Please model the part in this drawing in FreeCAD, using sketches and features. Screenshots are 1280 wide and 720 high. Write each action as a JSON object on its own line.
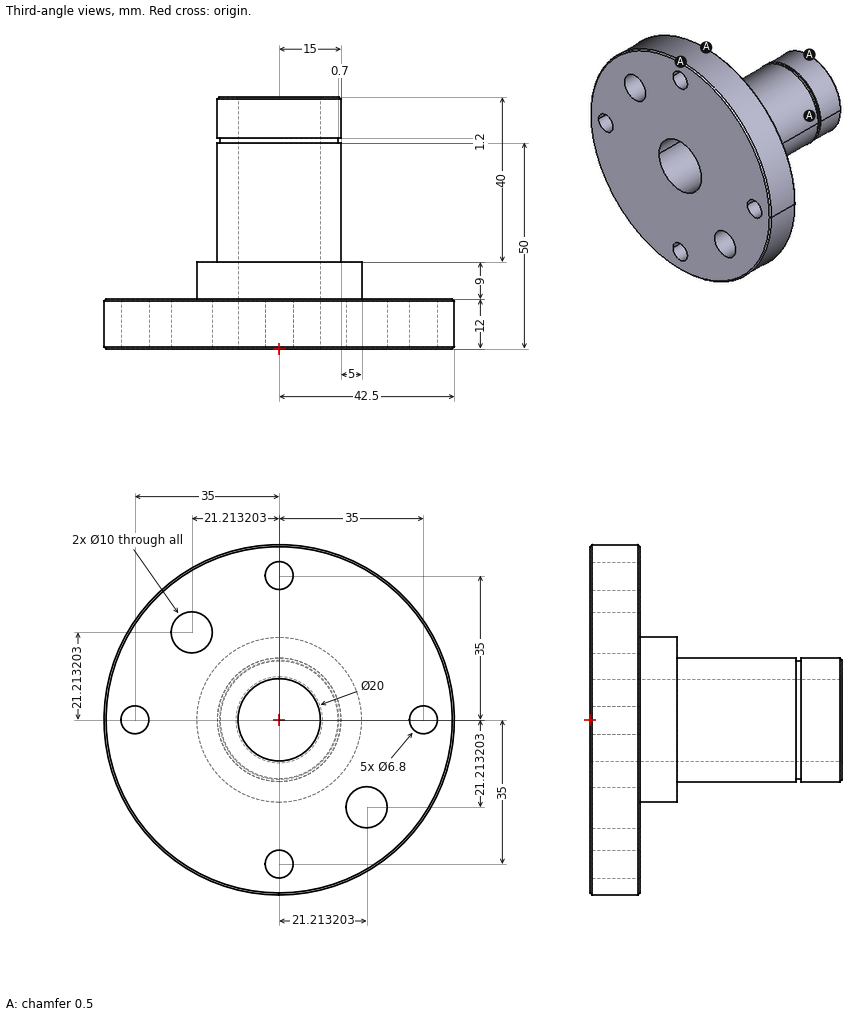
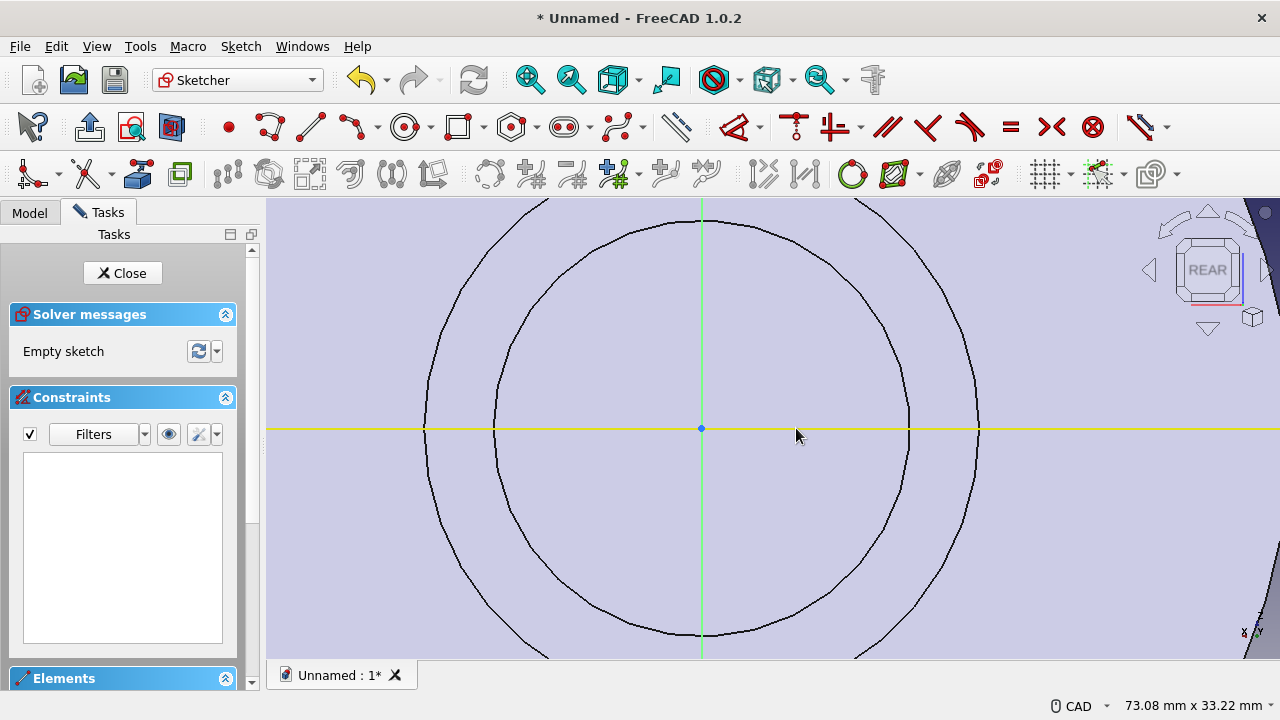
{"action": "left_click", "coordinate": [404, 128]}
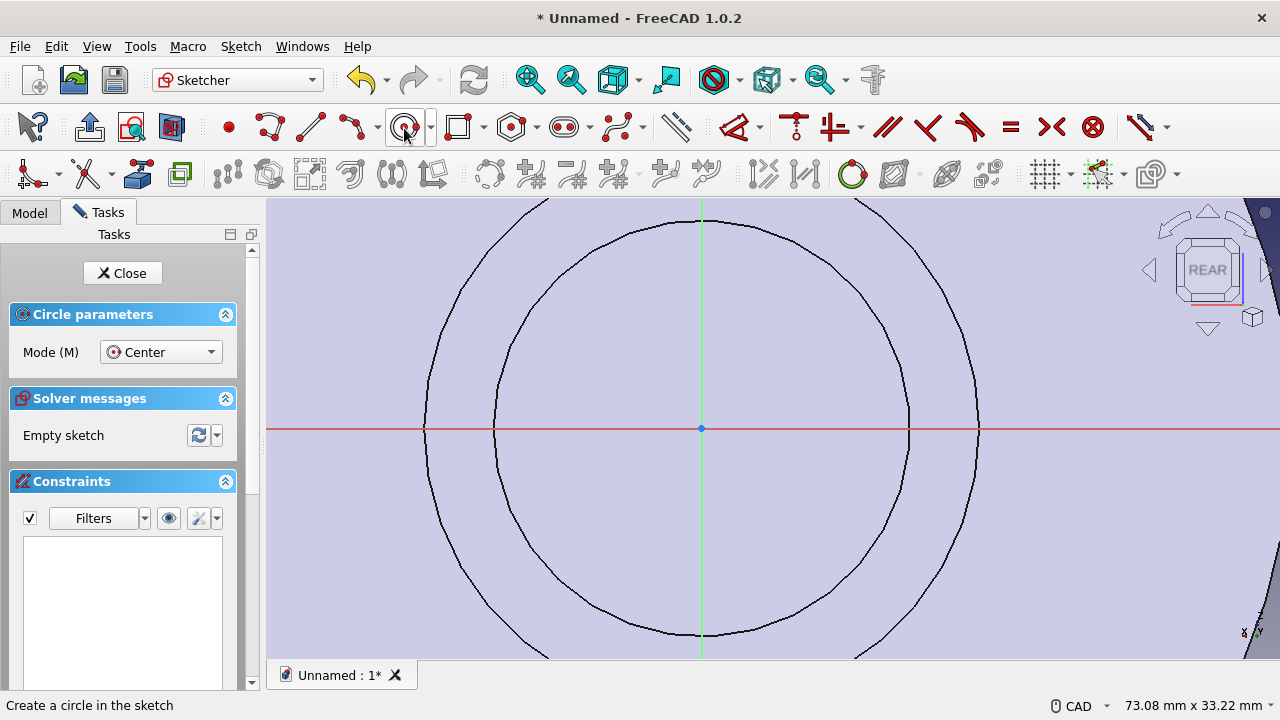
{"action": "left_click", "coordinate": [702, 428]}
{"action": "left_click", "coordinate": [800, 330]}
{"action": "key", "text": "Escape"}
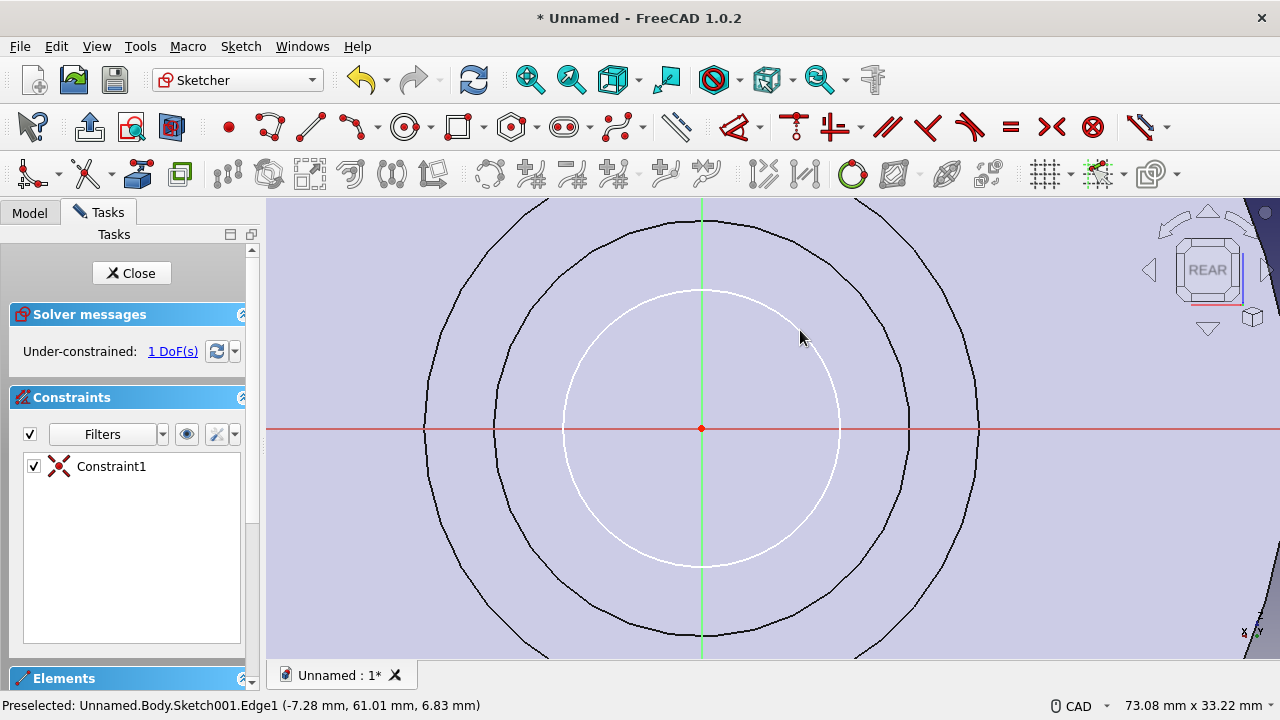
{"action": "left_click", "coordinate": [734, 128]}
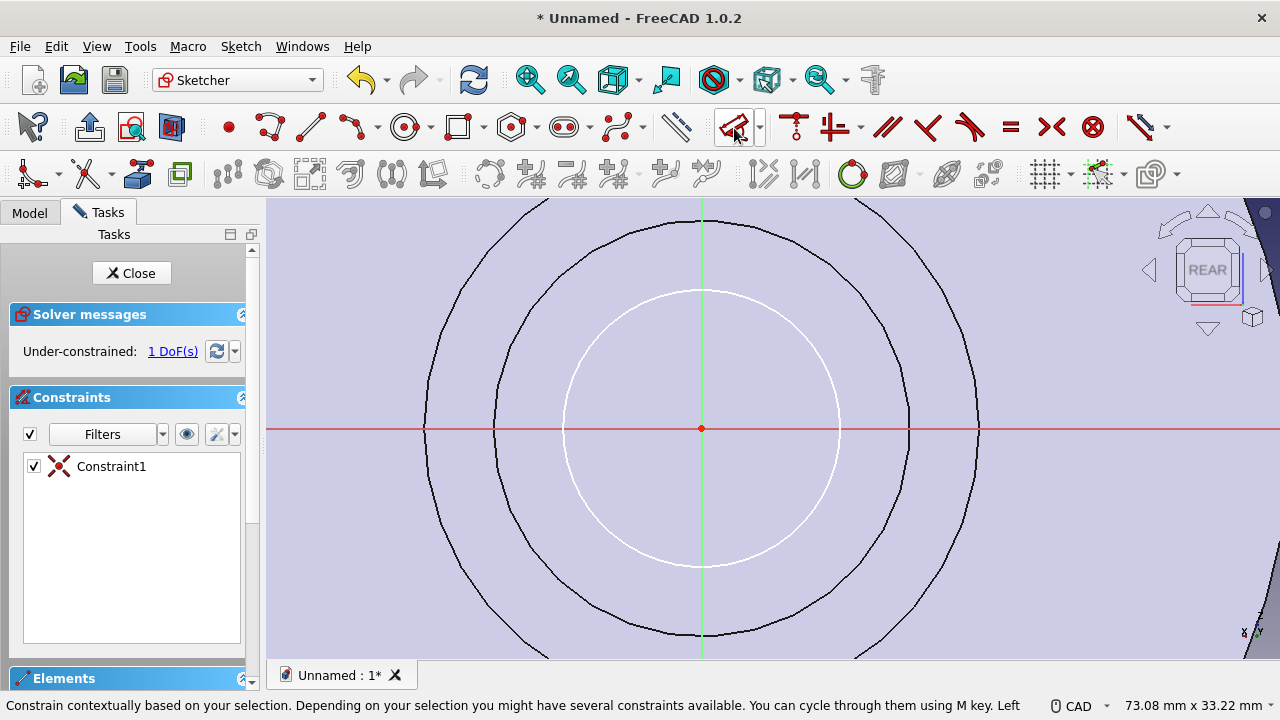
{"action": "left_click", "coordinate": [799, 330]}
{"action": "left_click", "coordinate": [821, 307]}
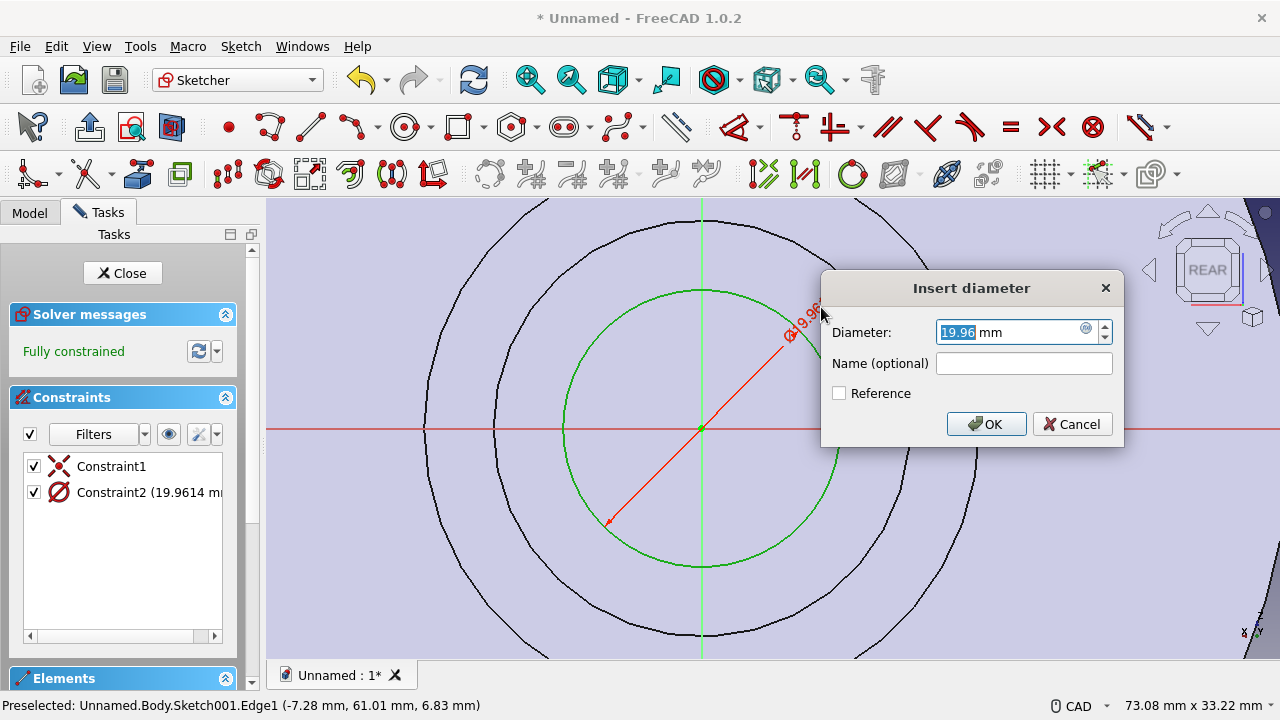
{"action": "type", "text": "20"}
{"action": "key", "text": "Return"}
{"action": "key", "text": "Escape"}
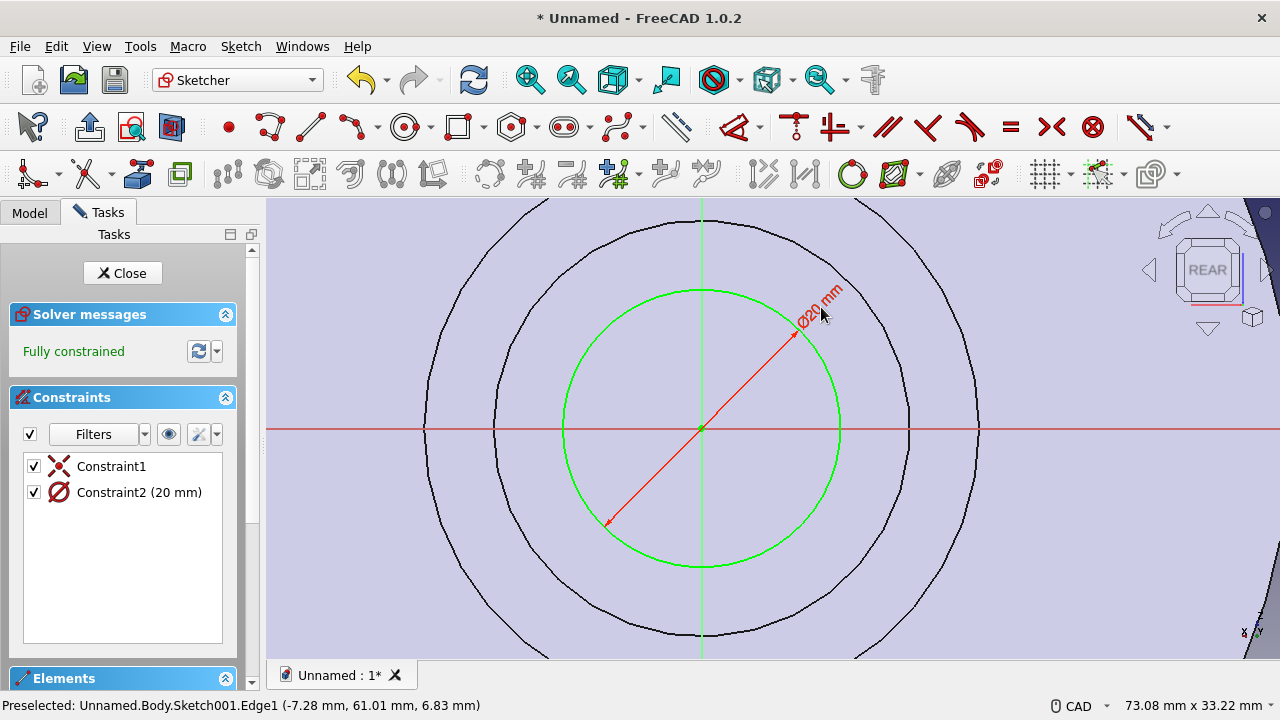
{"action": "left_click", "coordinate": [123, 273]}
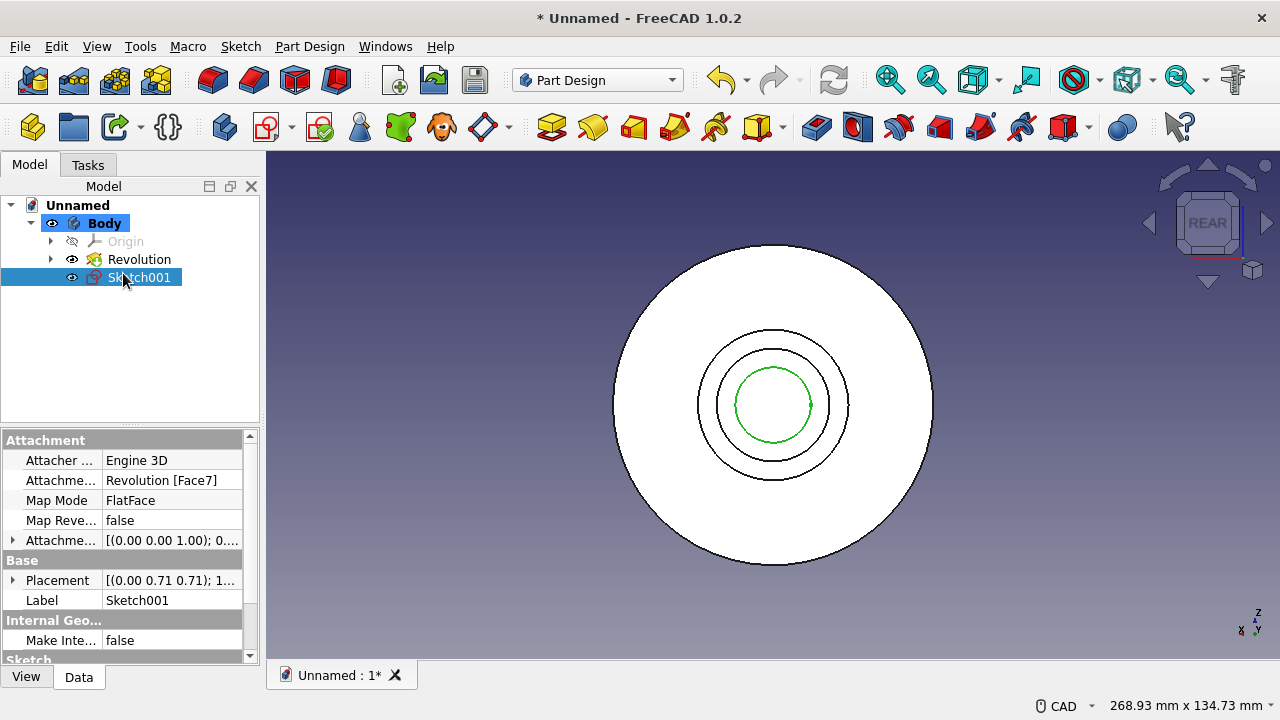
{"action": "left_click", "coordinate": [817, 128]}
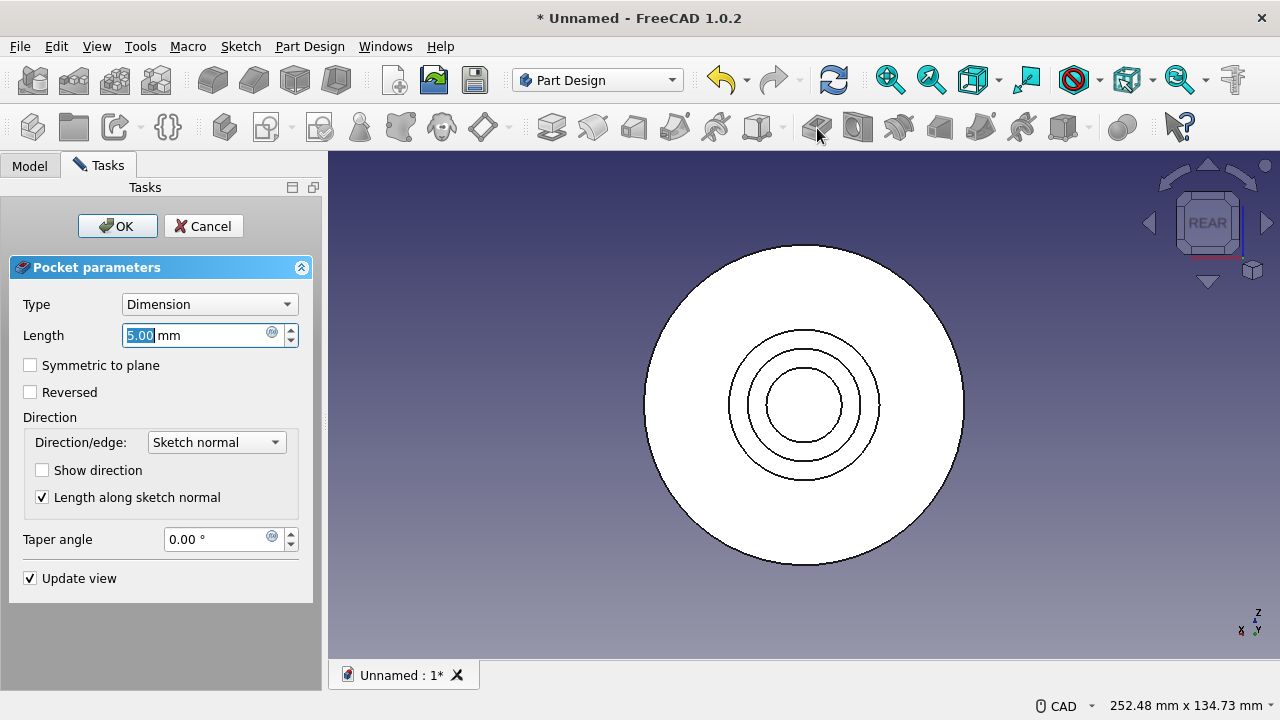
{"action": "left_click", "coordinate": [210, 304]}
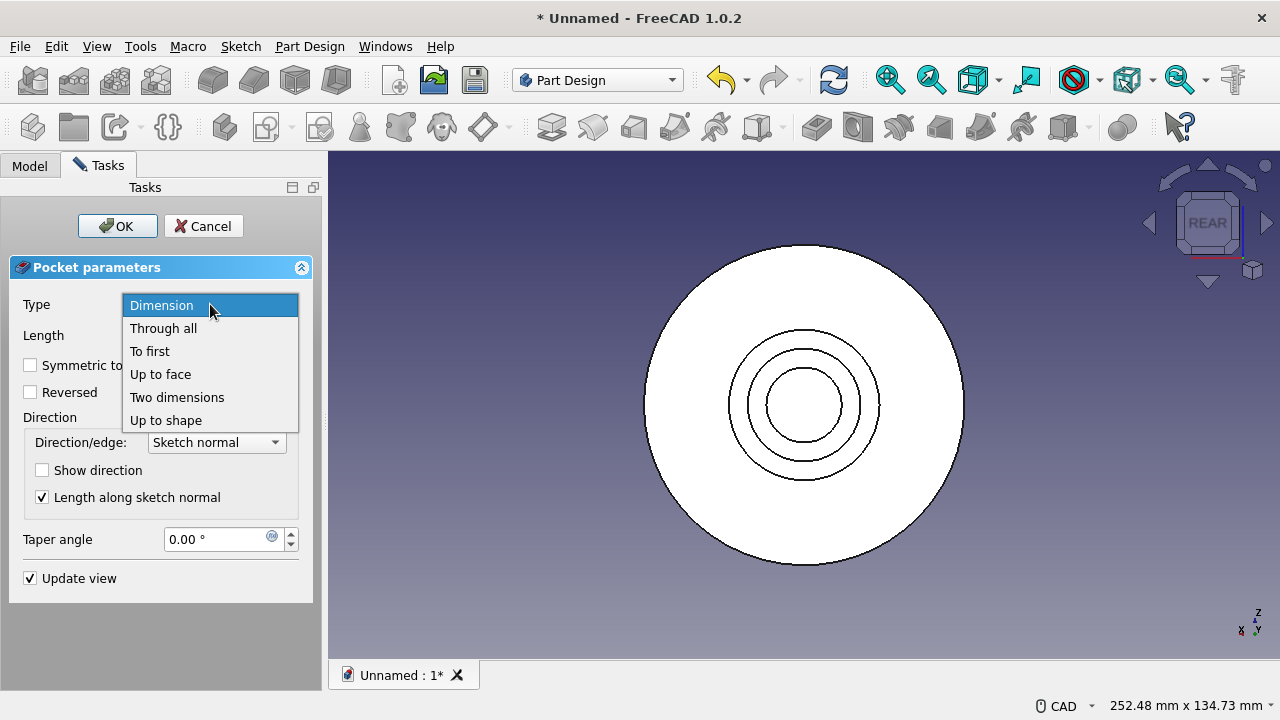
{"action": "left_click", "coordinate": [208, 328]}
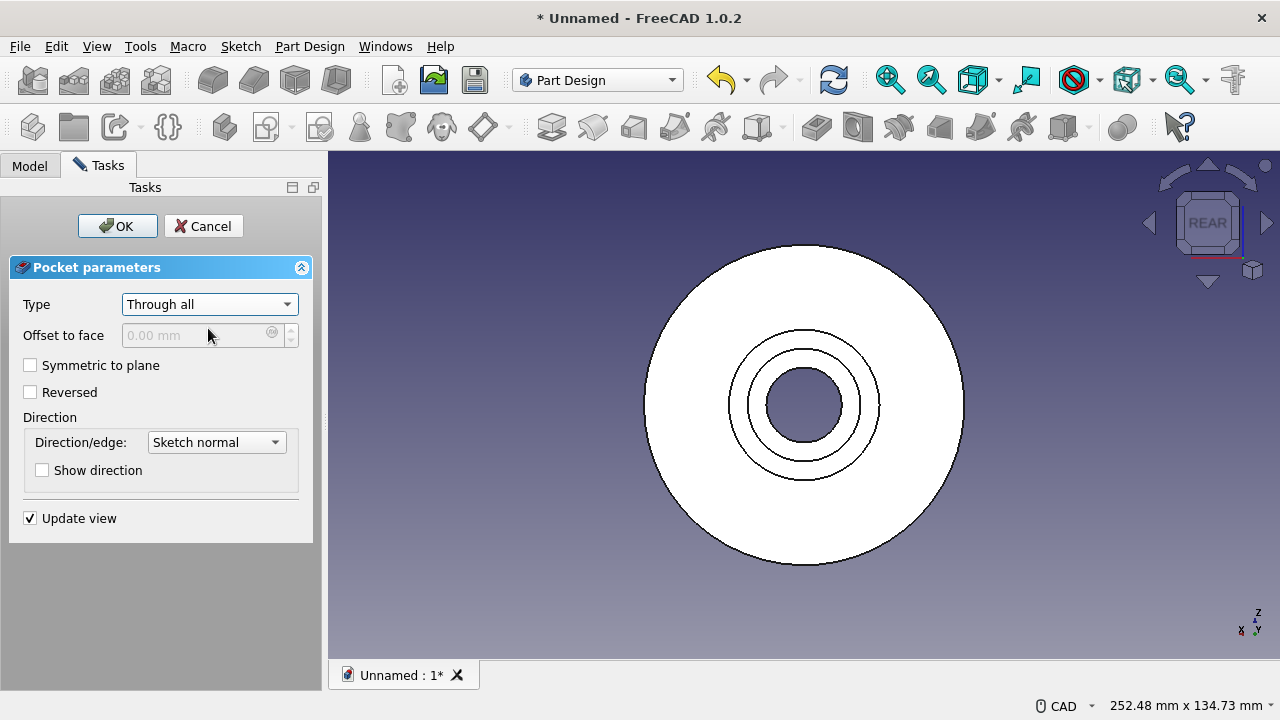
{"action": "left_click", "coordinate": [118, 226]}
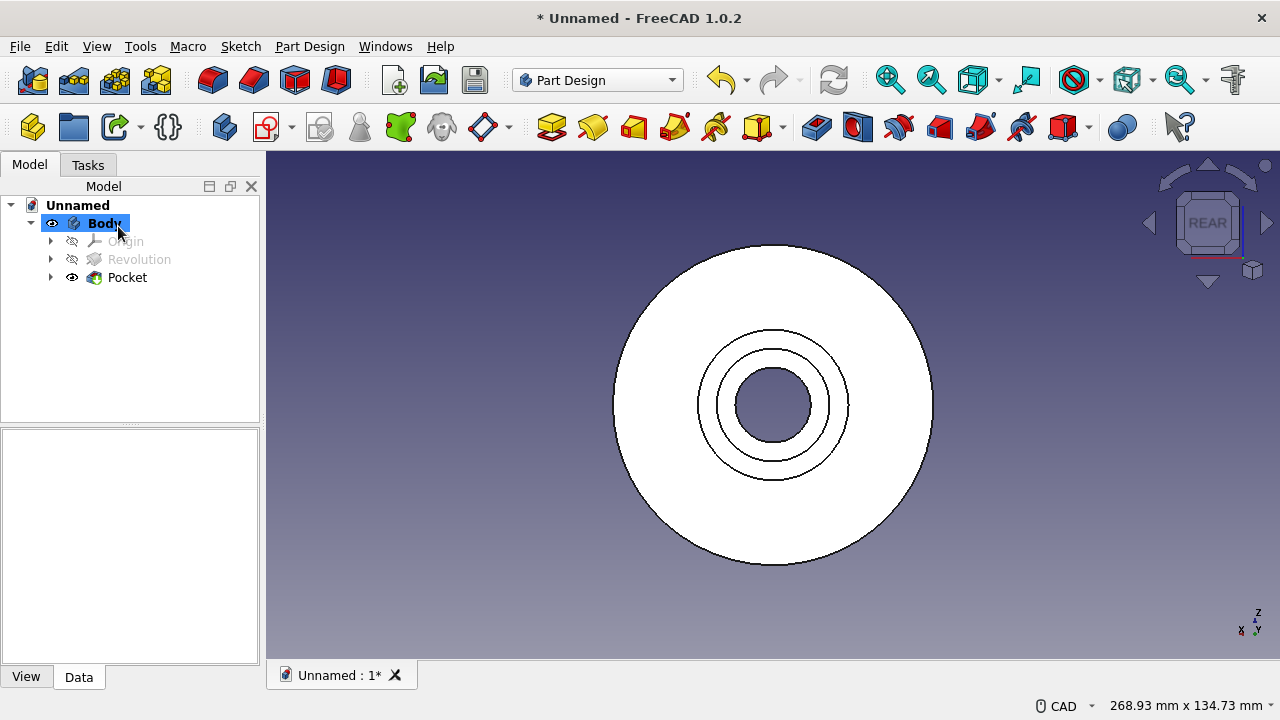
{"action": "left_click", "coordinate": [266, 128]}